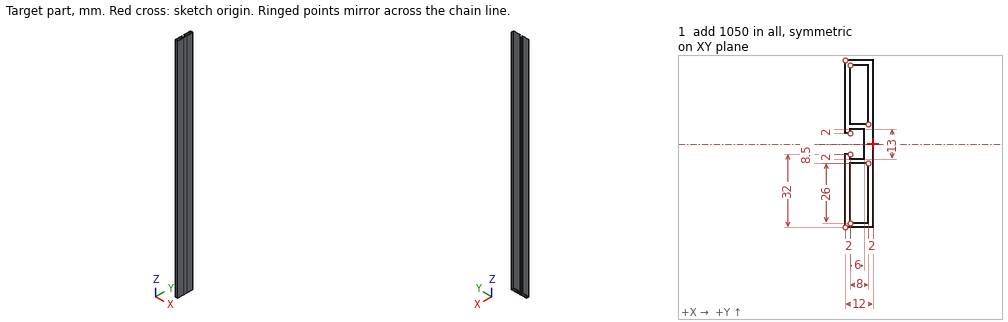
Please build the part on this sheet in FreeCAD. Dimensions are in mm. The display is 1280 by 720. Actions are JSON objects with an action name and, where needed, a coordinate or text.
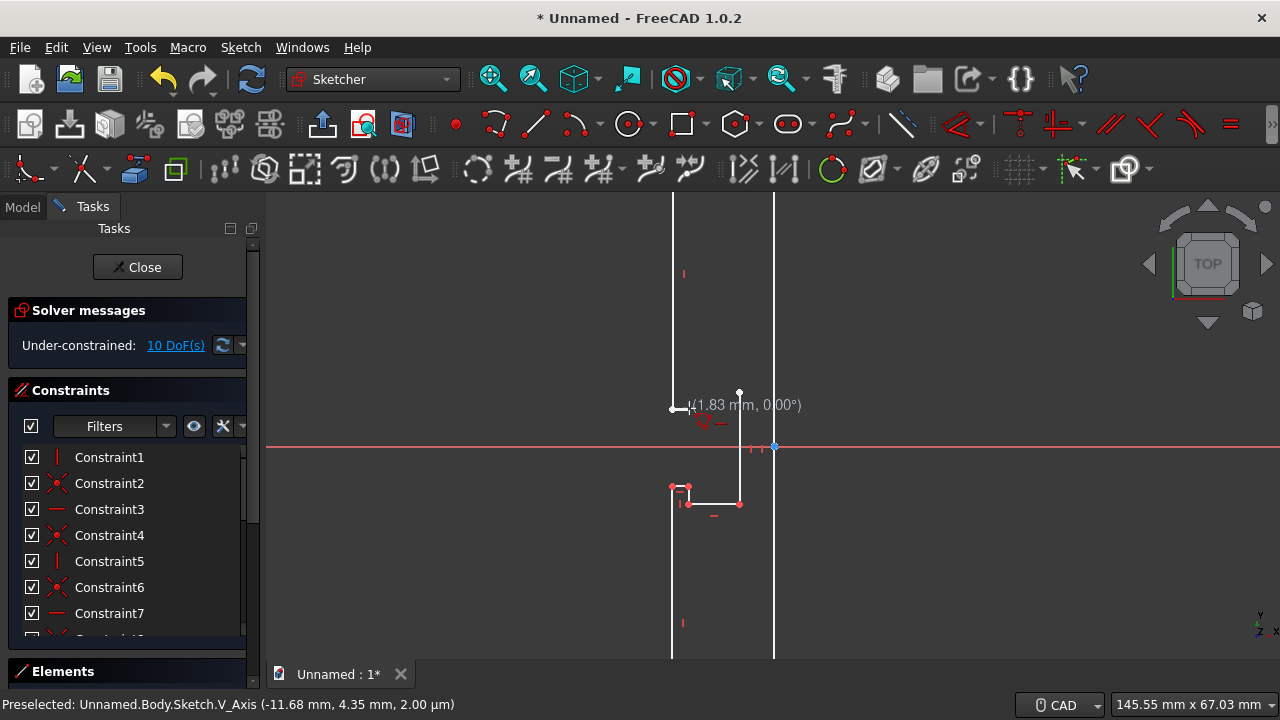
{"action": "left_click", "coordinate": [689, 407]}
{"action": "left_click", "coordinate": [689, 391]}
{"action": "left_click", "coordinate": [740, 393]}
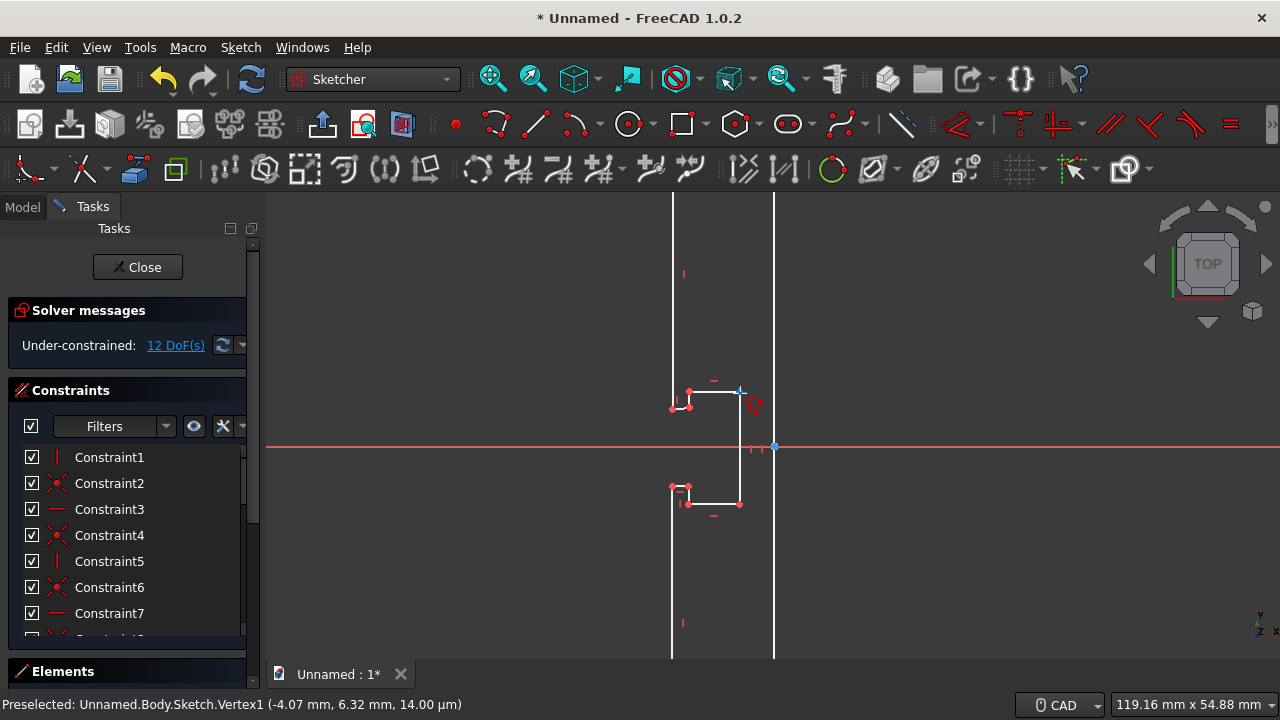
{"action": "left_click", "coordinate": [682, 124]}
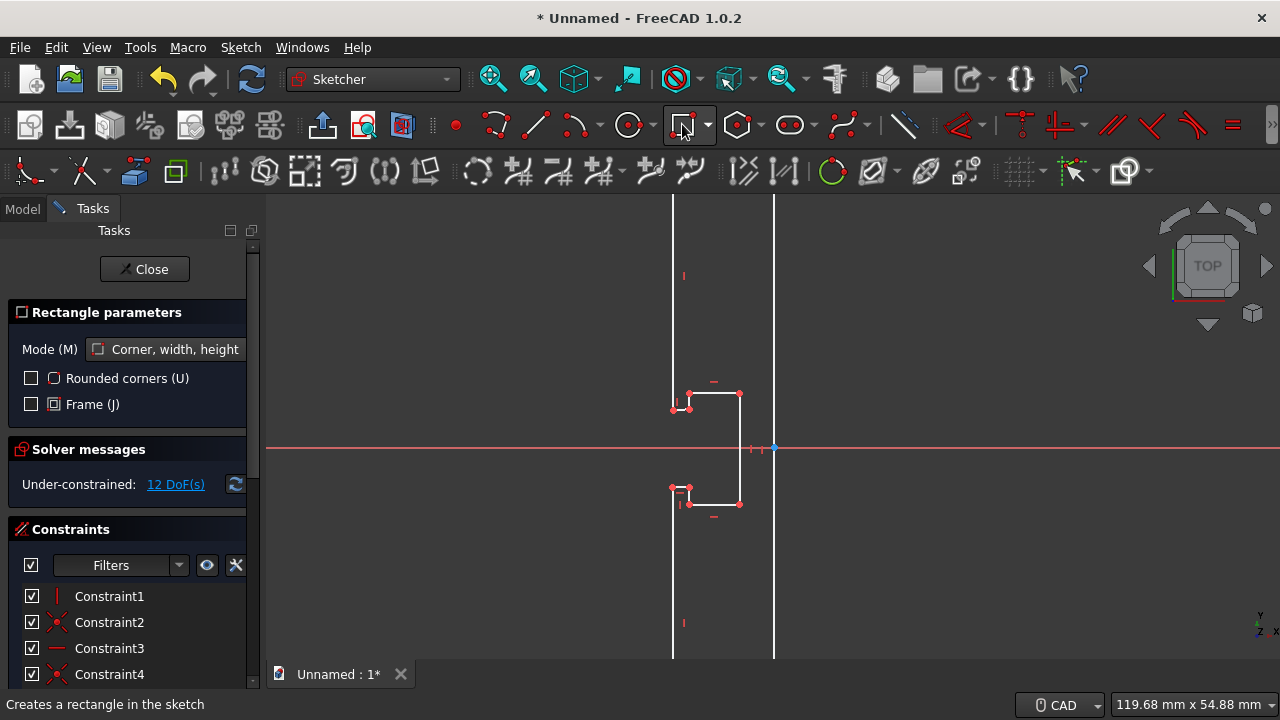
{"action": "left_click", "coordinate": [690, 520]}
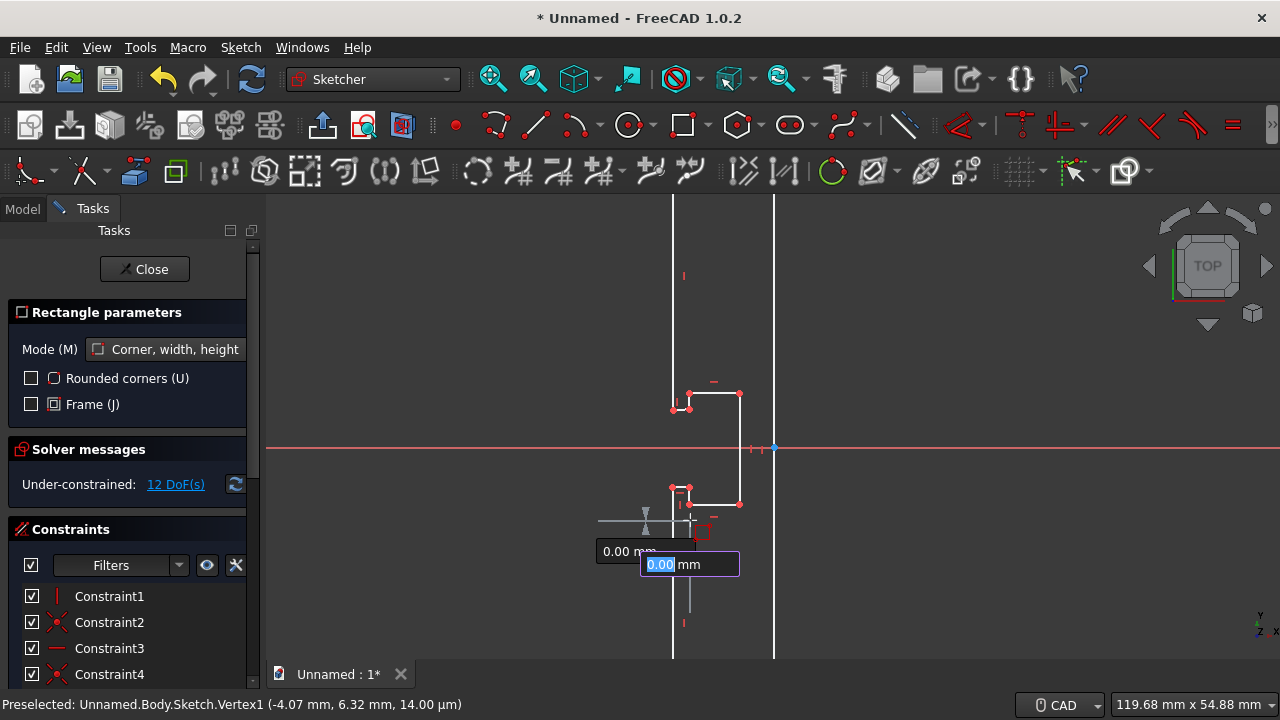
{"action": "scroll", "coordinate": [689, 409], "scroll_direction": "down", "scroll_amount": 4}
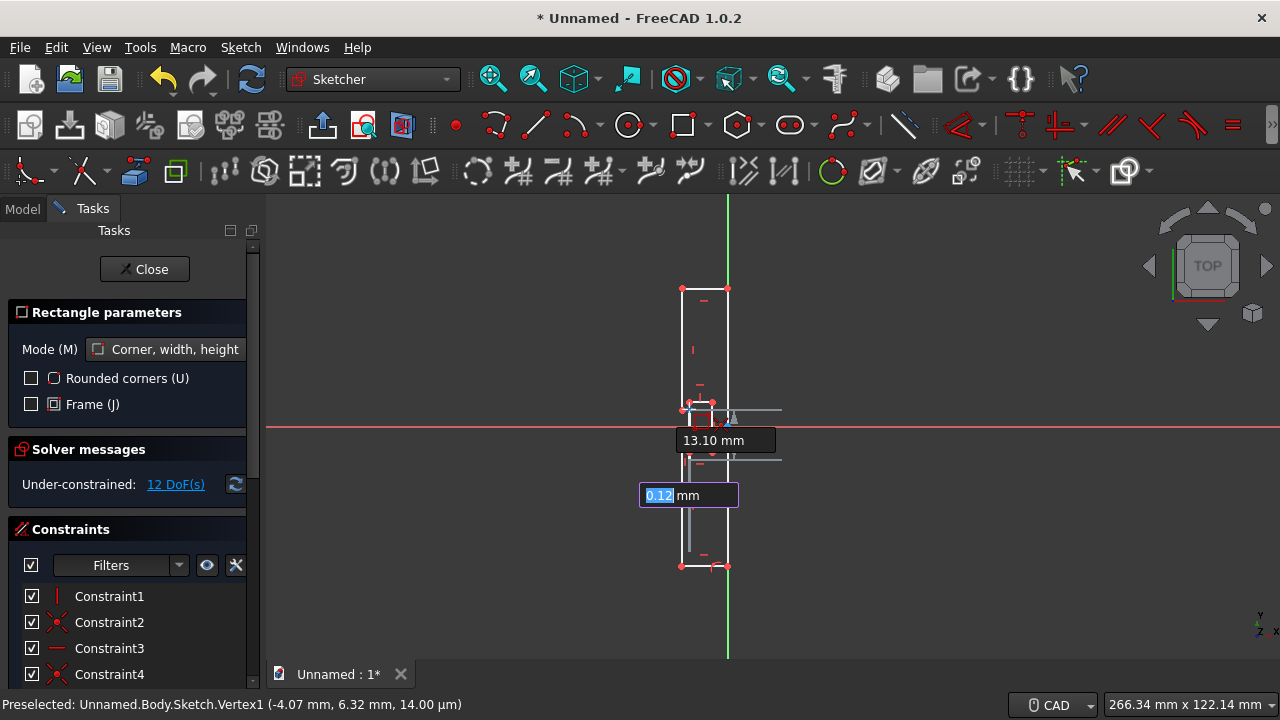
{"action": "scroll", "coordinate": [720, 558], "scroll_direction": "up", "scroll_amount": 4}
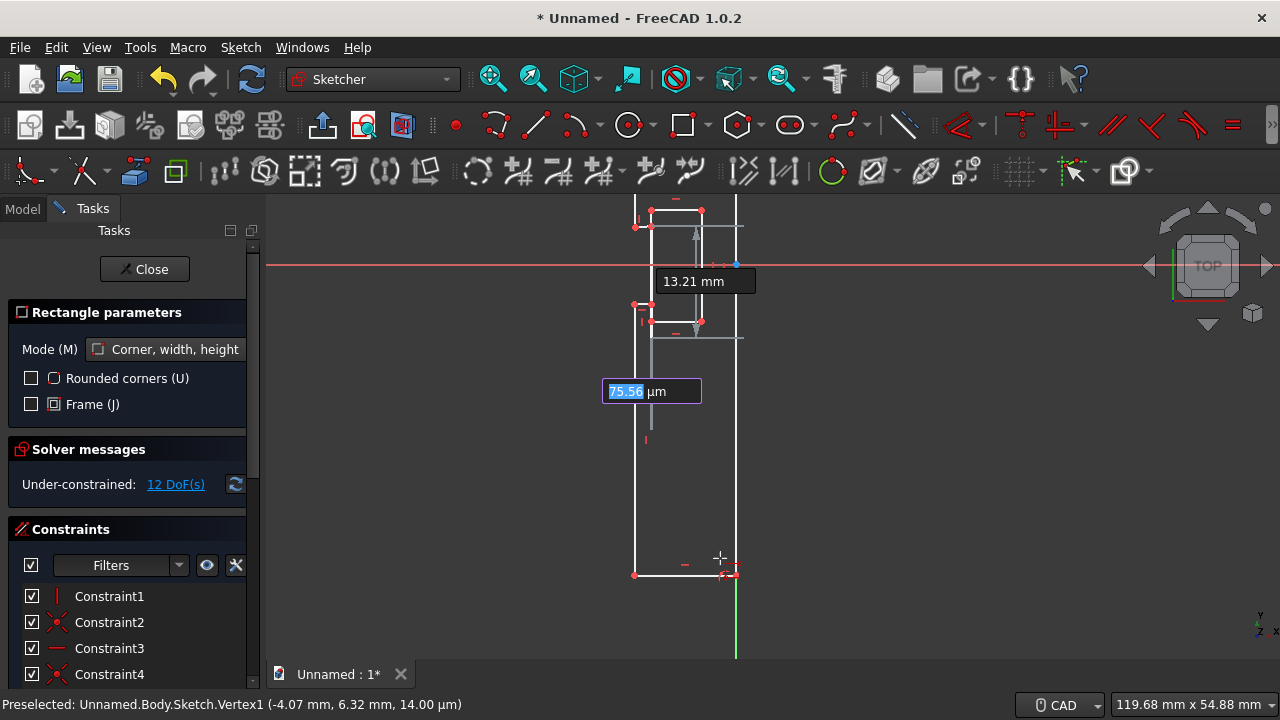
{"action": "left_click", "coordinate": [719, 557]}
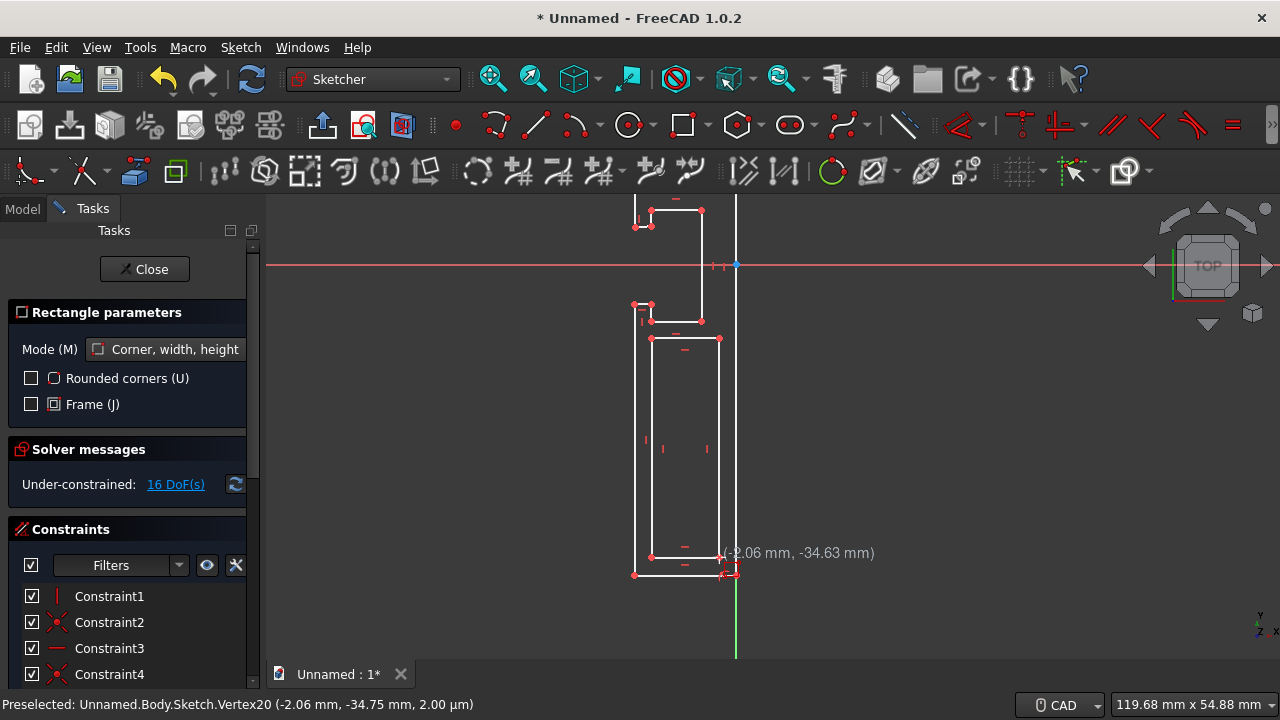
{"action": "scroll", "coordinate": [720, 559], "scroll_direction": "down", "scroll_amount": 4}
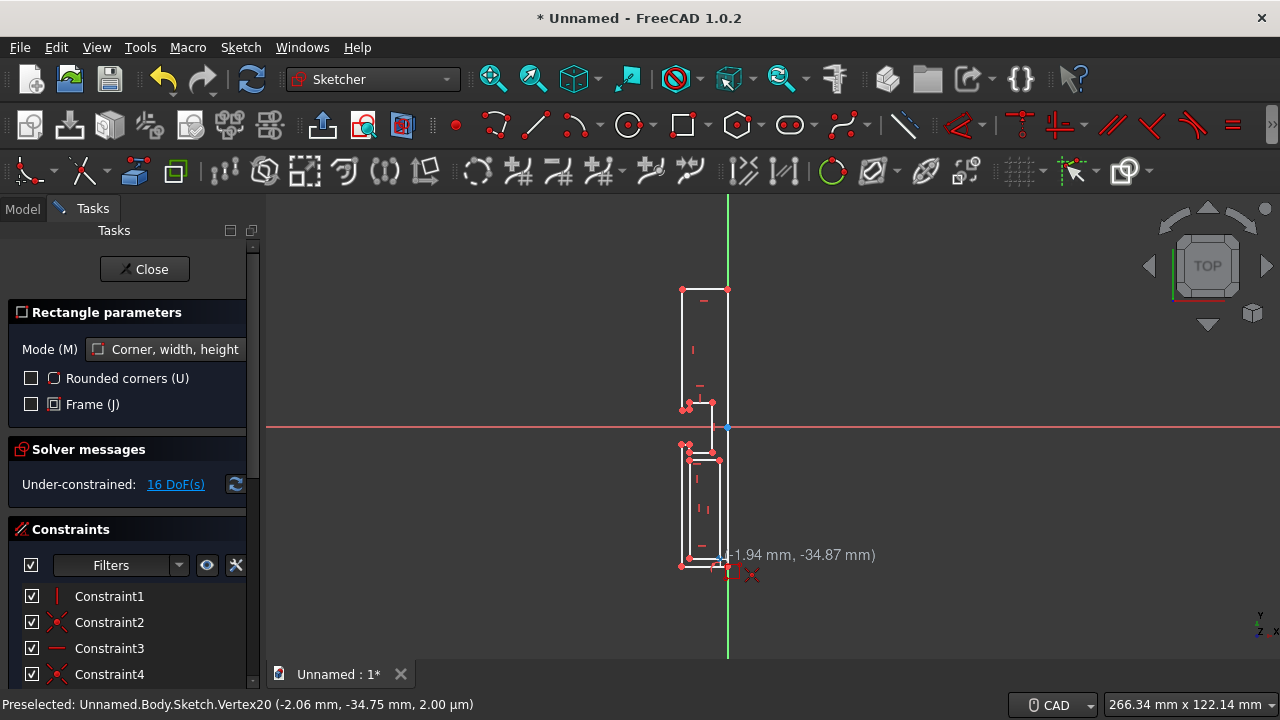
{"action": "scroll", "coordinate": [690, 296], "scroll_direction": "up", "scroll_amount": 4}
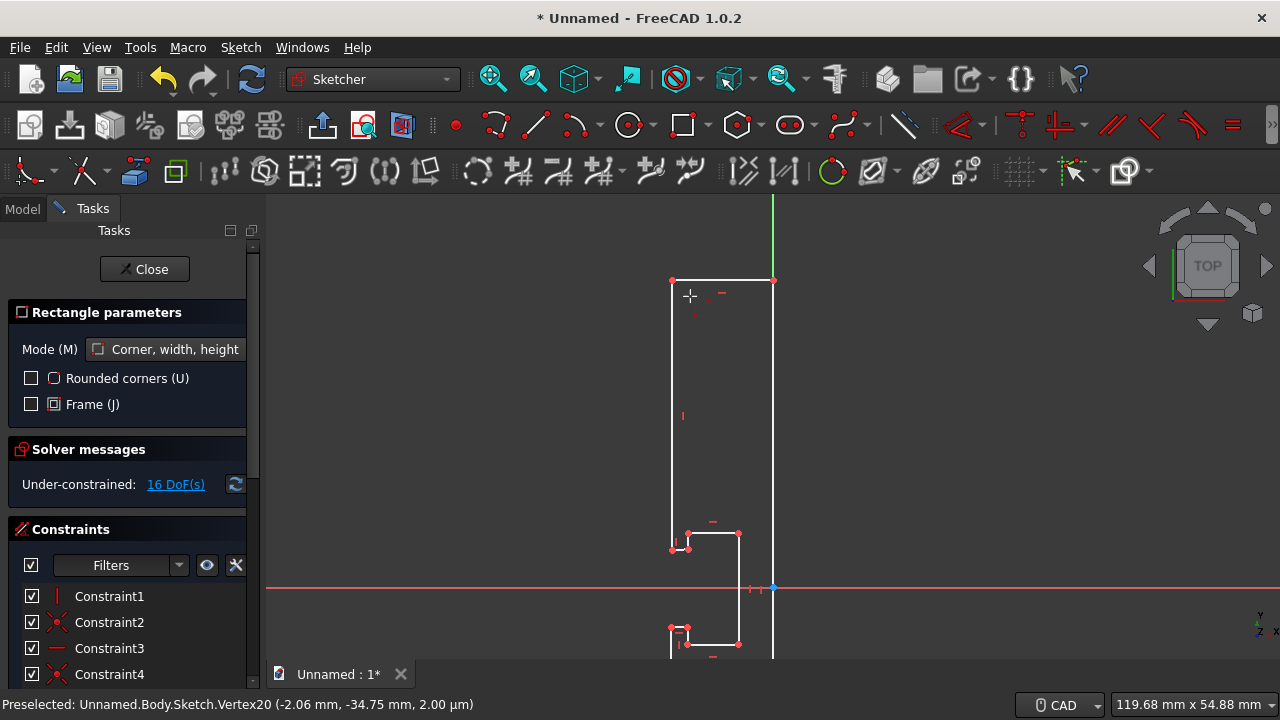
{"action": "left_click", "coordinate": [689, 295]}
{"action": "left_click", "coordinate": [756, 516]}
{"action": "key", "text": "Escape"}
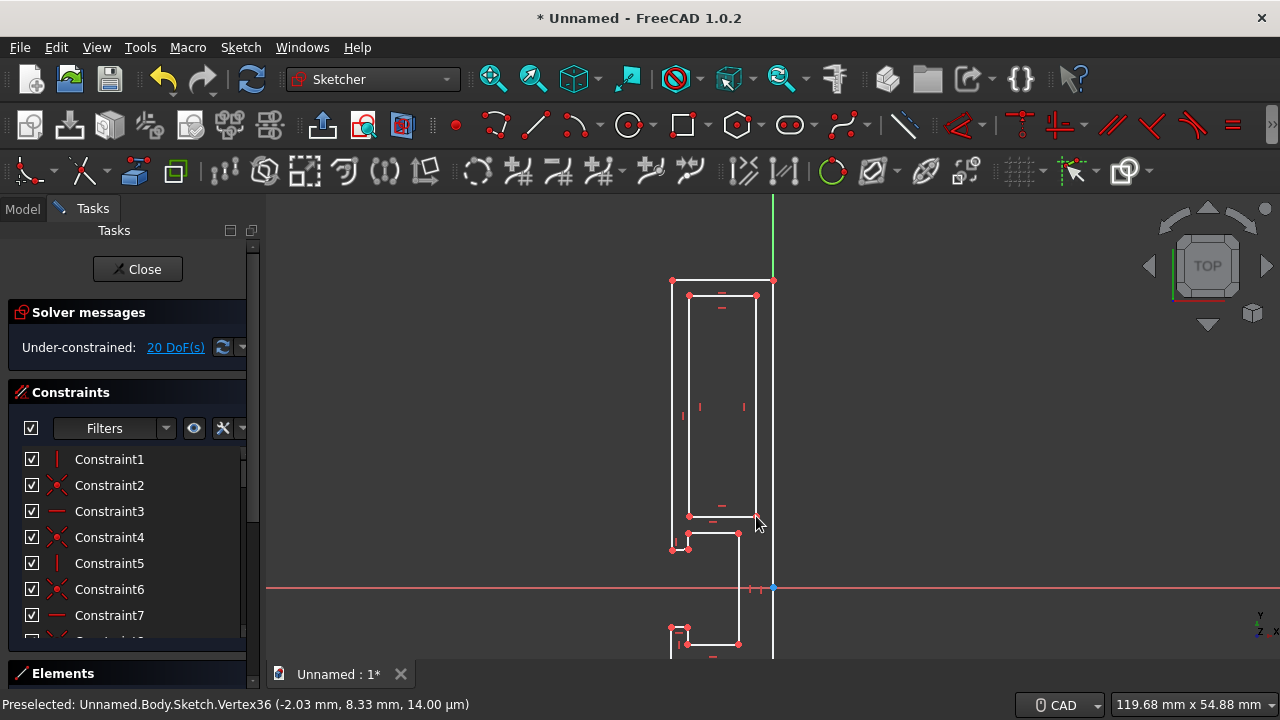
{"action": "scroll", "coordinate": [680, 550], "scroll_direction": "up", "scroll_amount": 3}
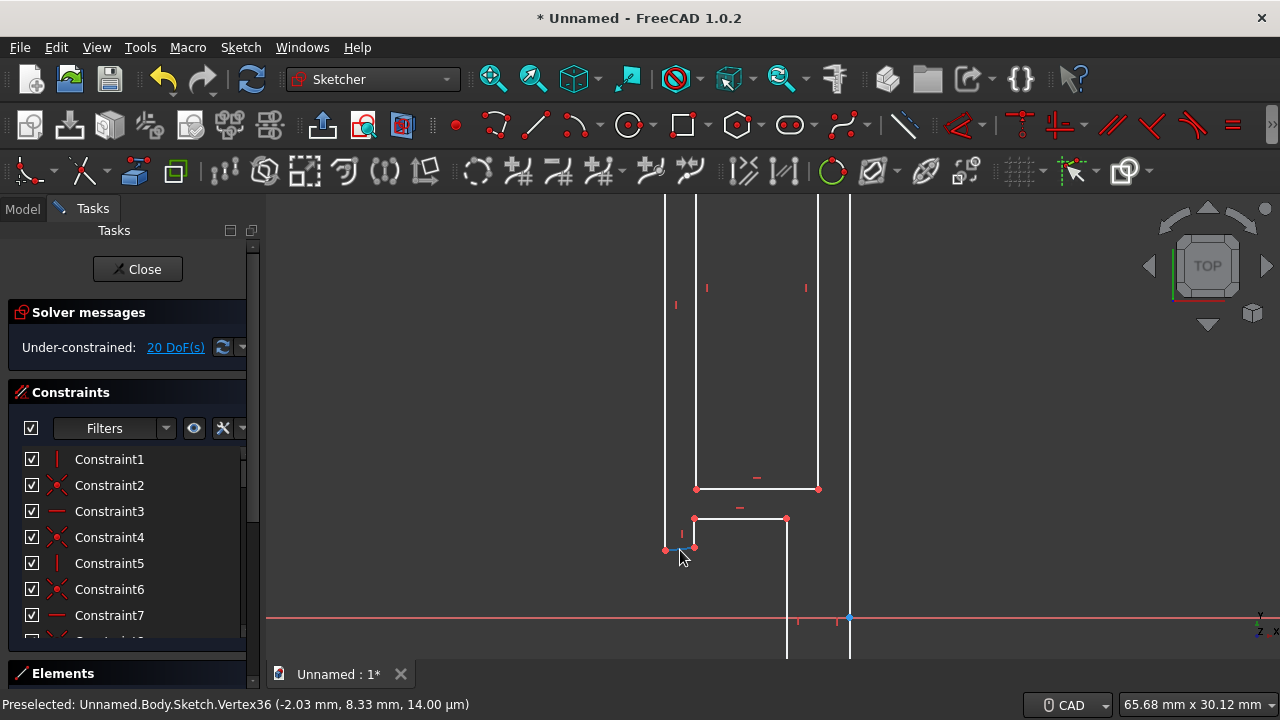
{"action": "left_click", "coordinate": [680, 549]}